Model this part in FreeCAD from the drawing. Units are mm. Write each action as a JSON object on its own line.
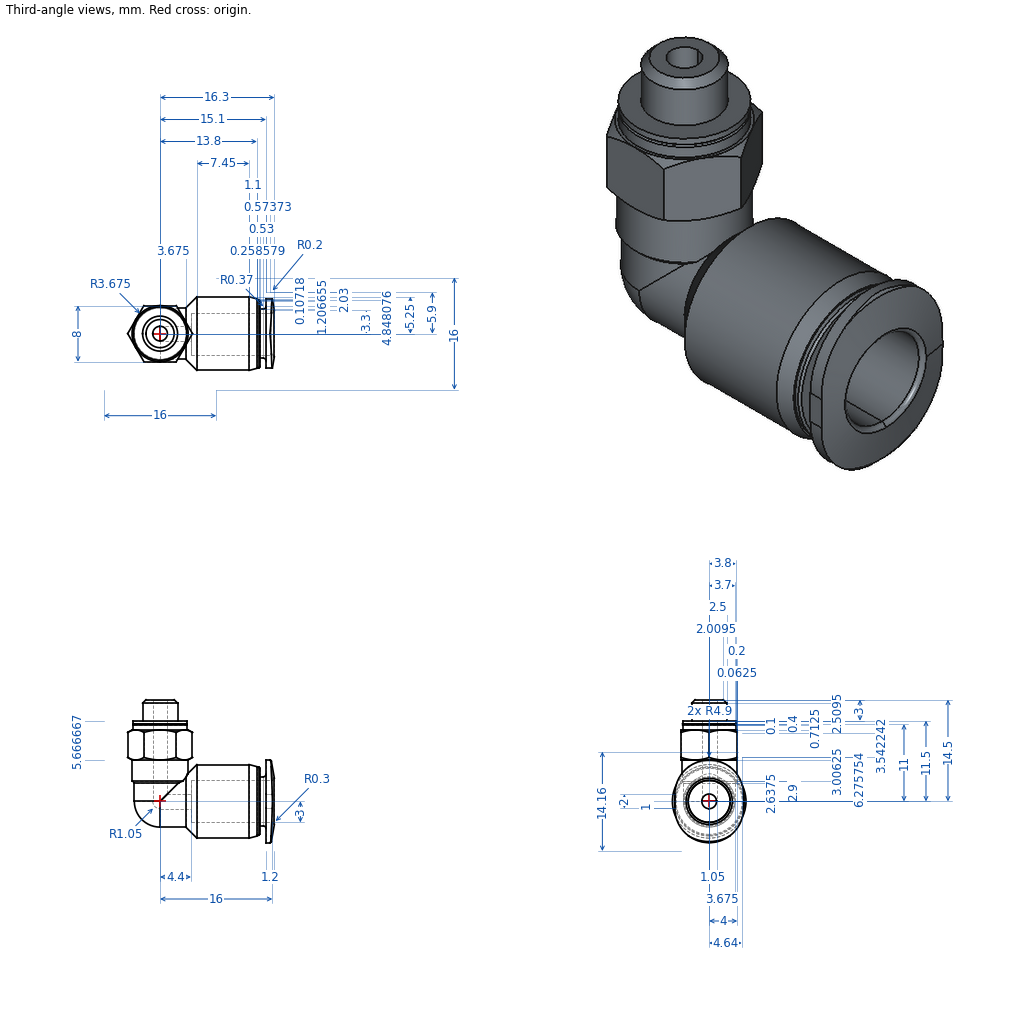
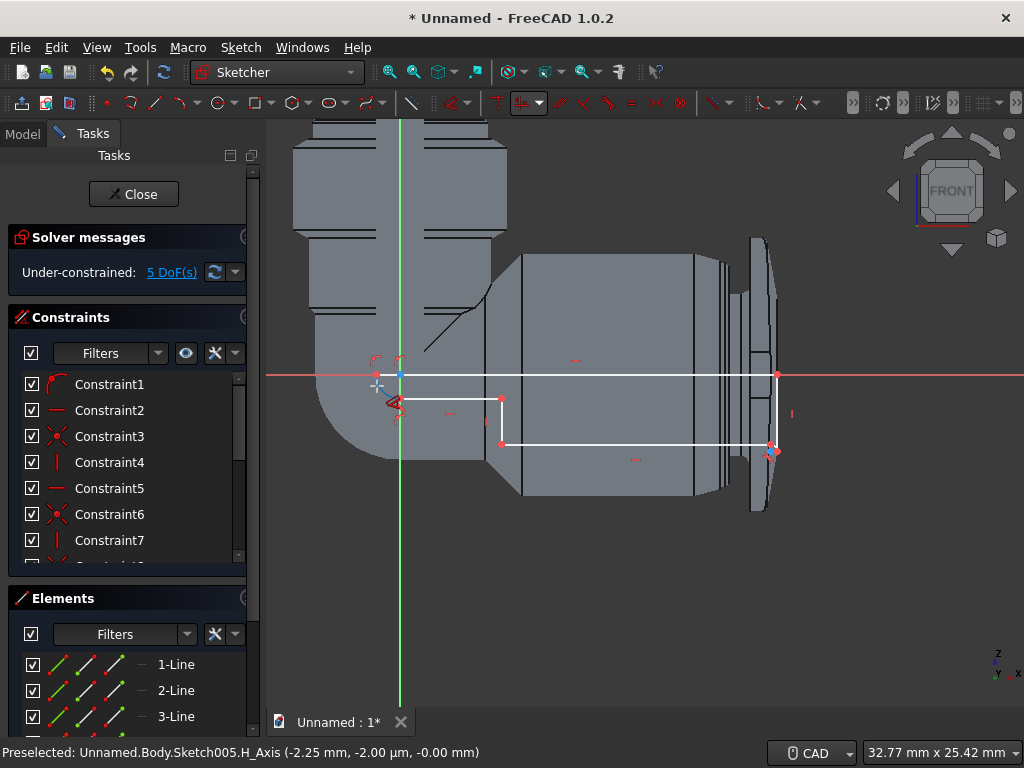
{"action": "scroll", "coordinate": [774, 445], "scroll_direction": "up", "scroll_amount": 9}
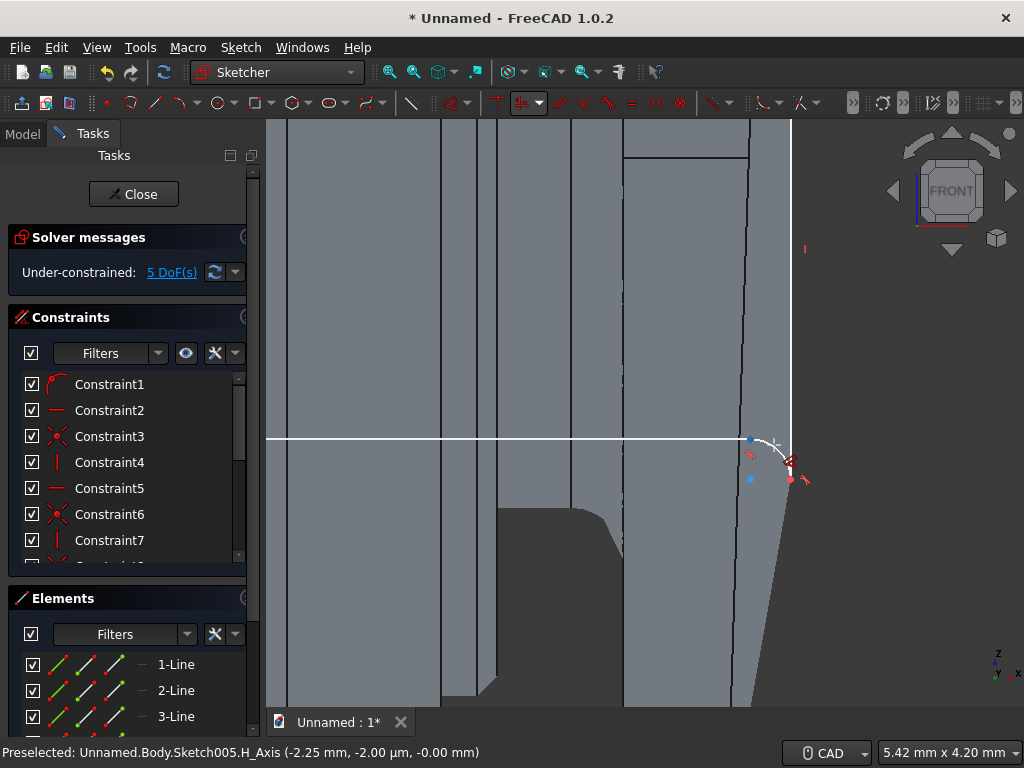
{"action": "left_click", "coordinate": [769, 444]}
{"action": "left_click", "coordinate": [810, 439]}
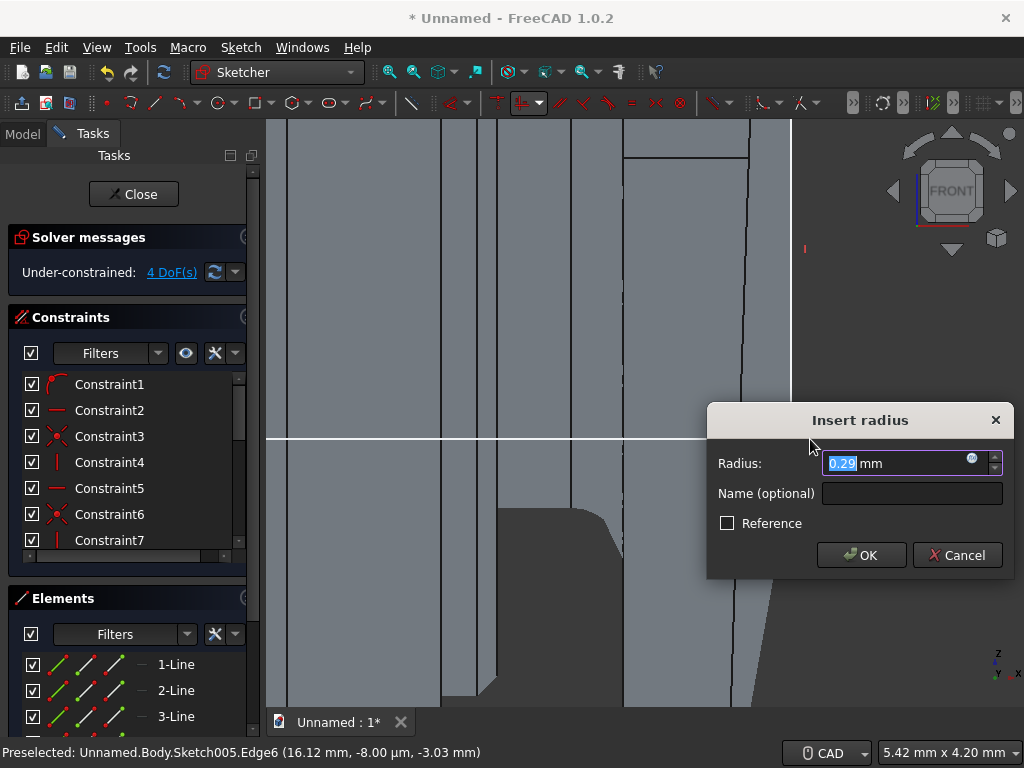
{"action": "type", "text": "0.3"}
{"action": "key", "text": "Return"}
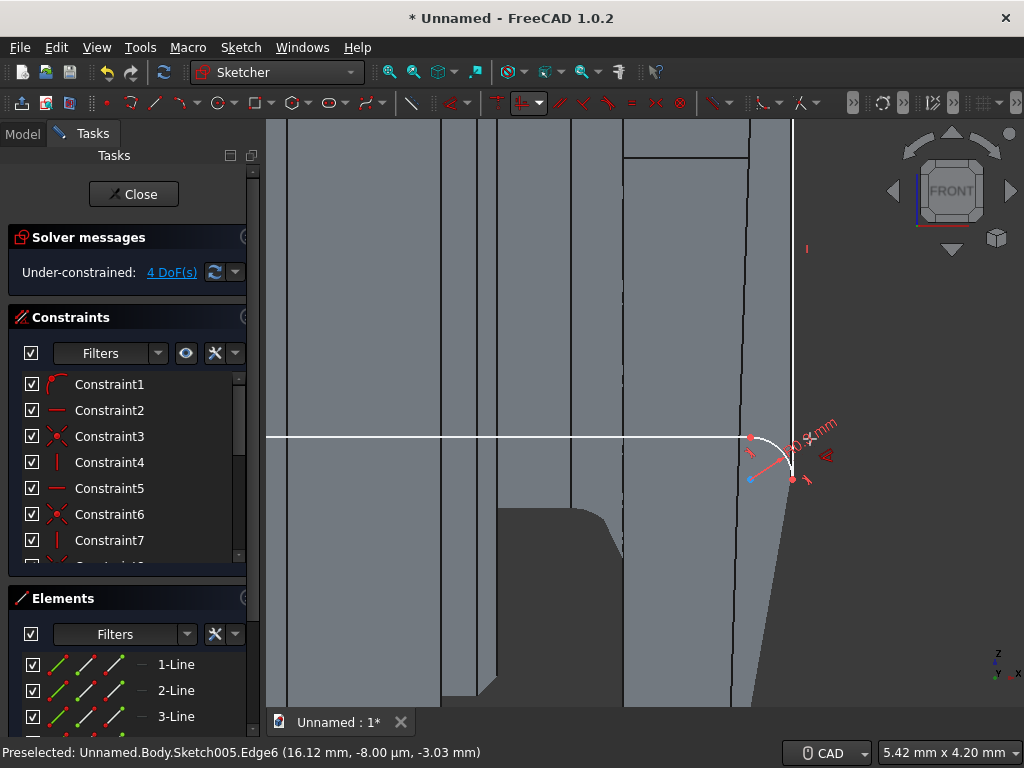
{"action": "scroll", "coordinate": [774, 445], "scroll_direction": "down", "scroll_amount": 9}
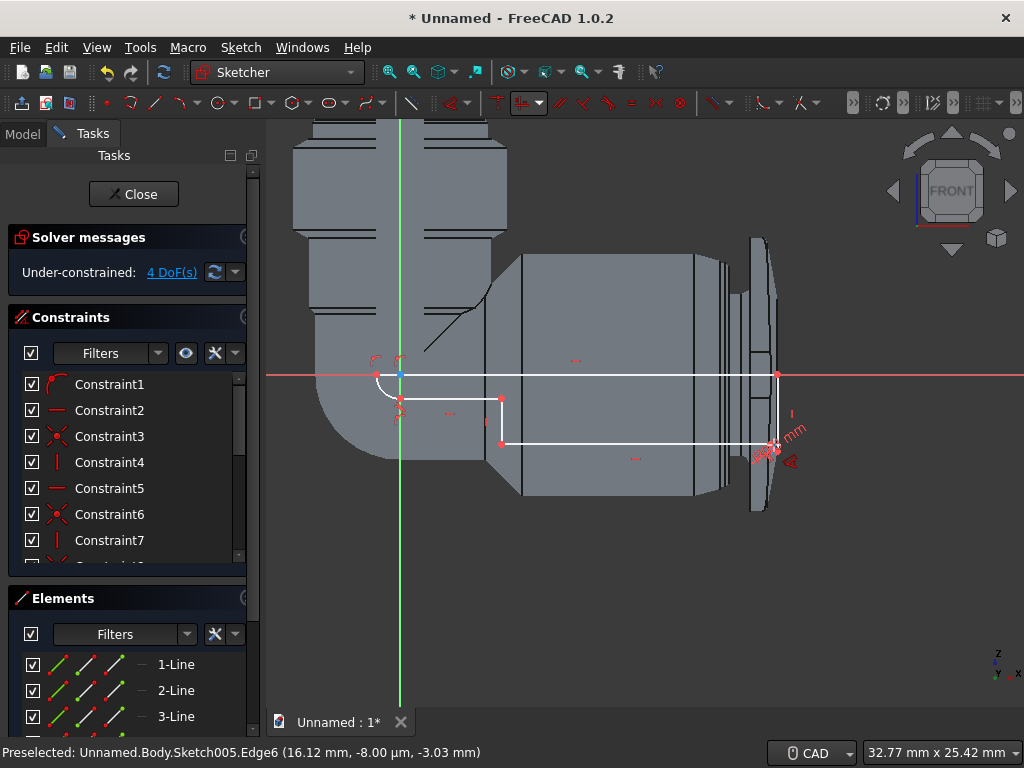
{"action": "scroll", "coordinate": [379, 386], "scroll_direction": "up", "scroll_amount": 3}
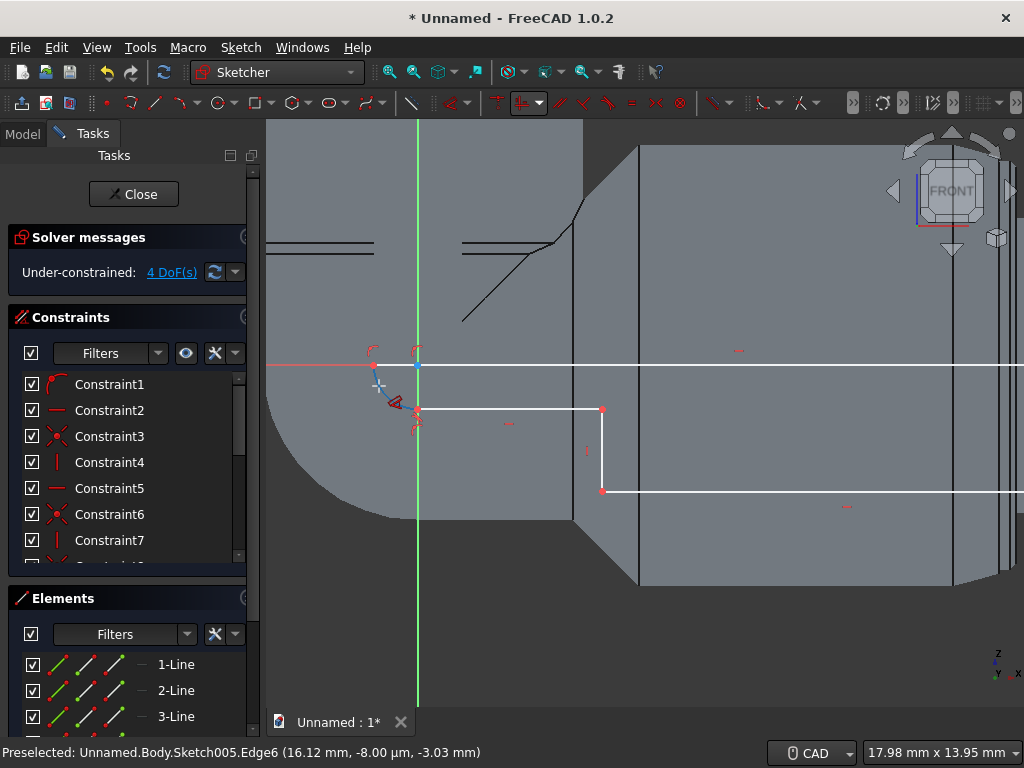
{"action": "left_click", "coordinate": [379, 385]}
{"action": "left_click", "coordinate": [350, 399]}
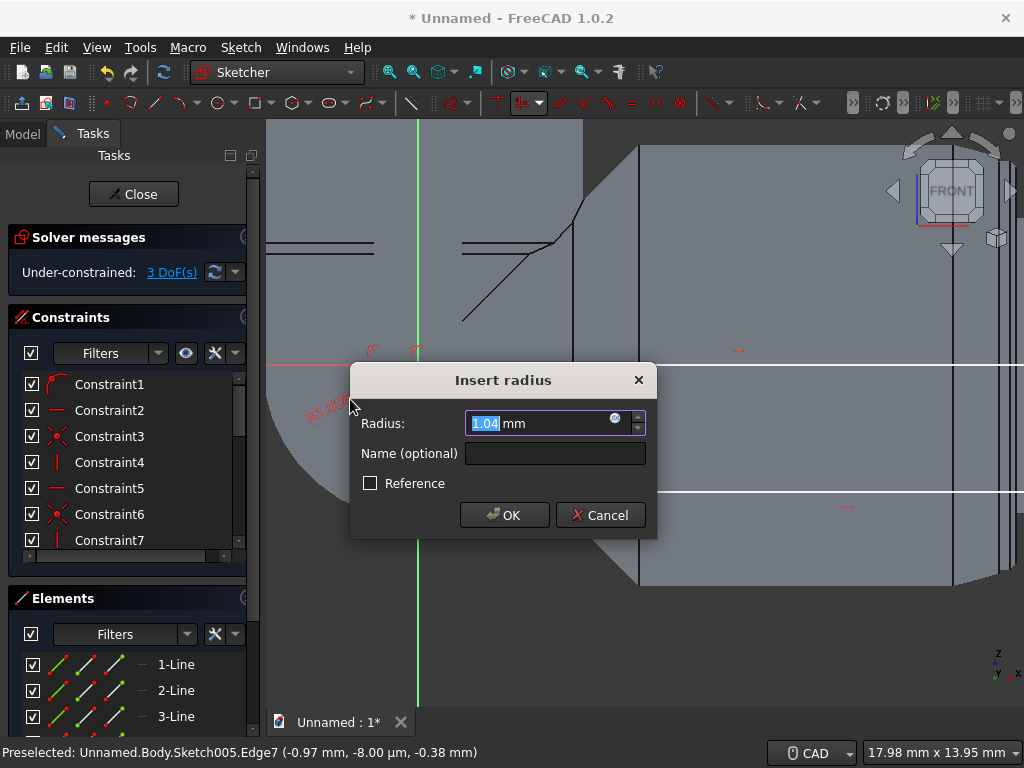
{"action": "type", "text": "1.05"}
{"action": "key", "text": "Return"}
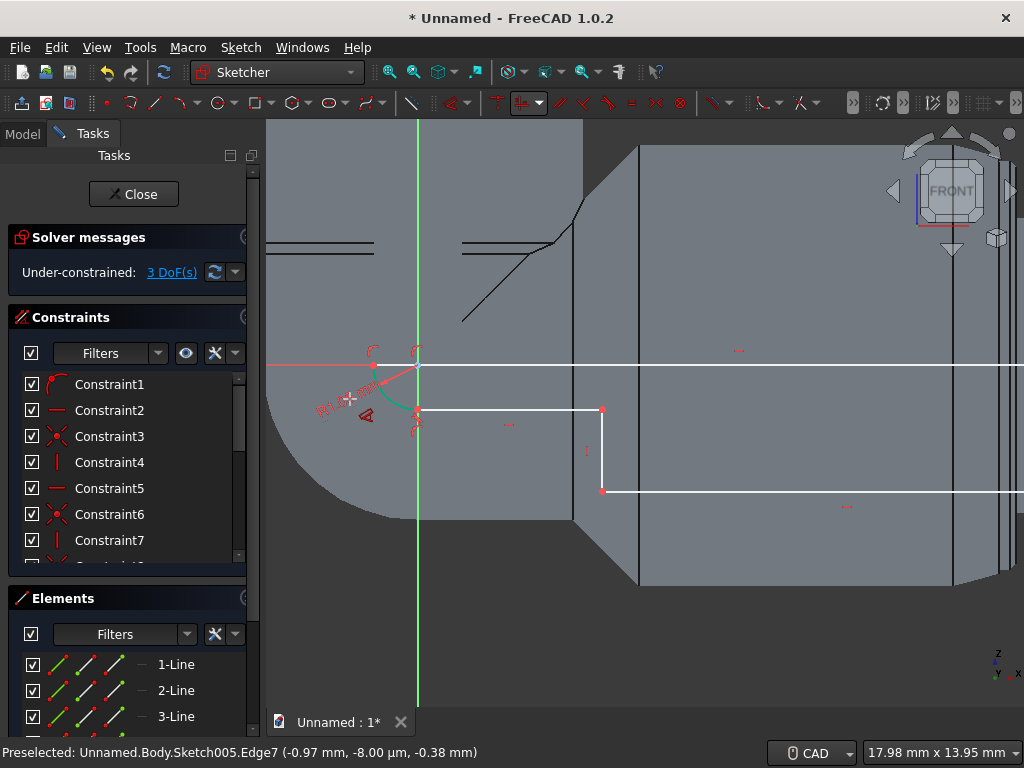
{"action": "scroll", "coordinate": [379, 386], "scroll_direction": "down", "scroll_amount": 3}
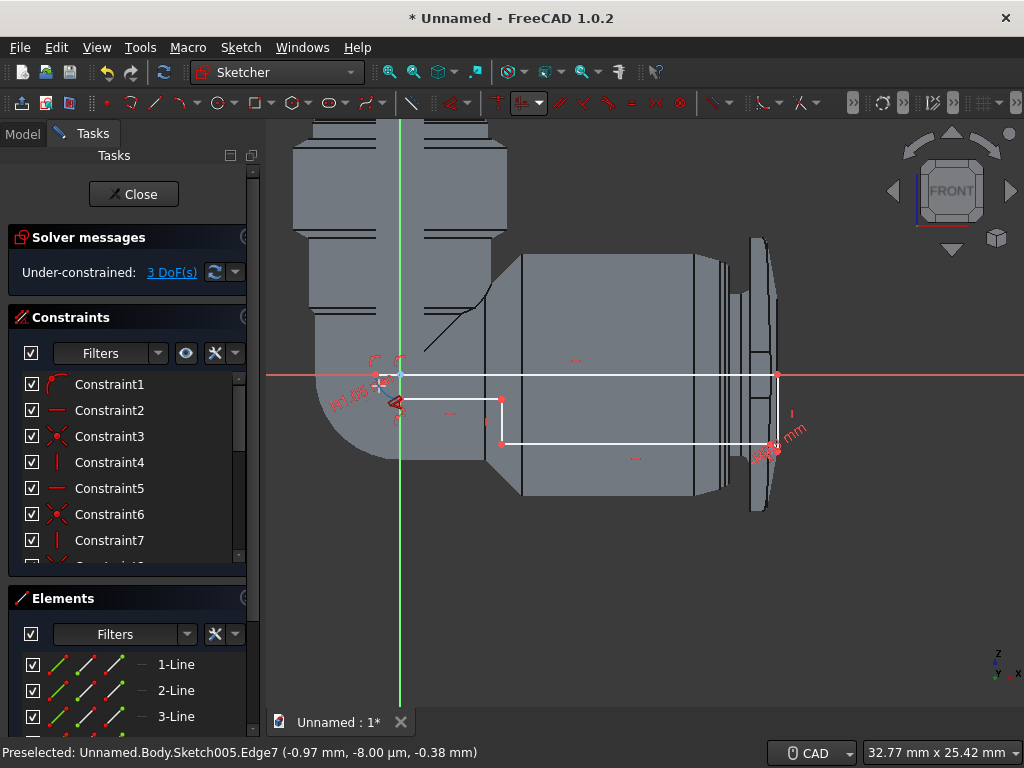
{"action": "scroll", "coordinate": [771, 444], "scroll_direction": "up", "scroll_amount": 3}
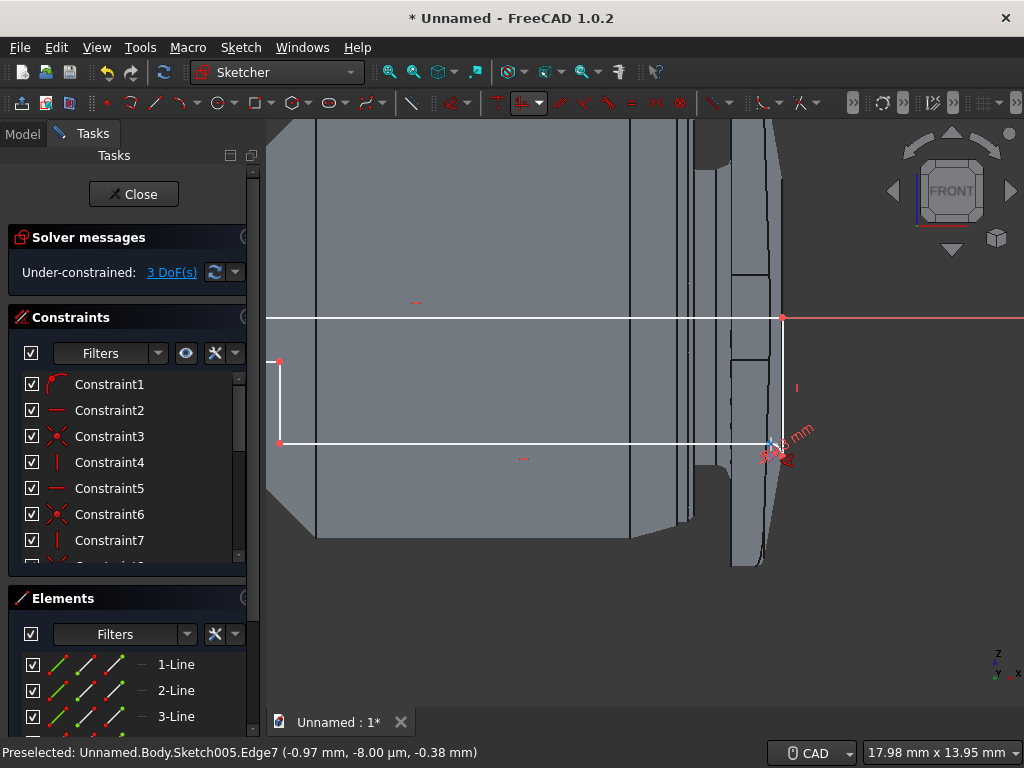
{"action": "left_click", "coordinate": [770, 444]}
{"action": "left_click", "coordinate": [804, 381]}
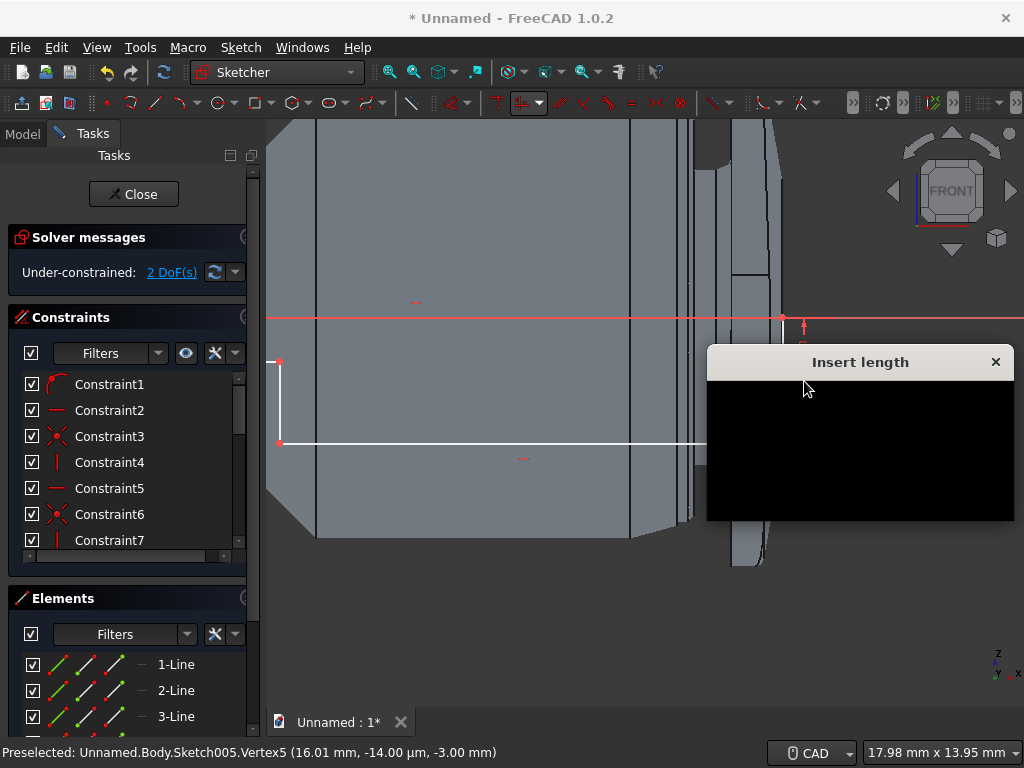
{"action": "type", "text": "3"}
{"action": "key", "text": "Return"}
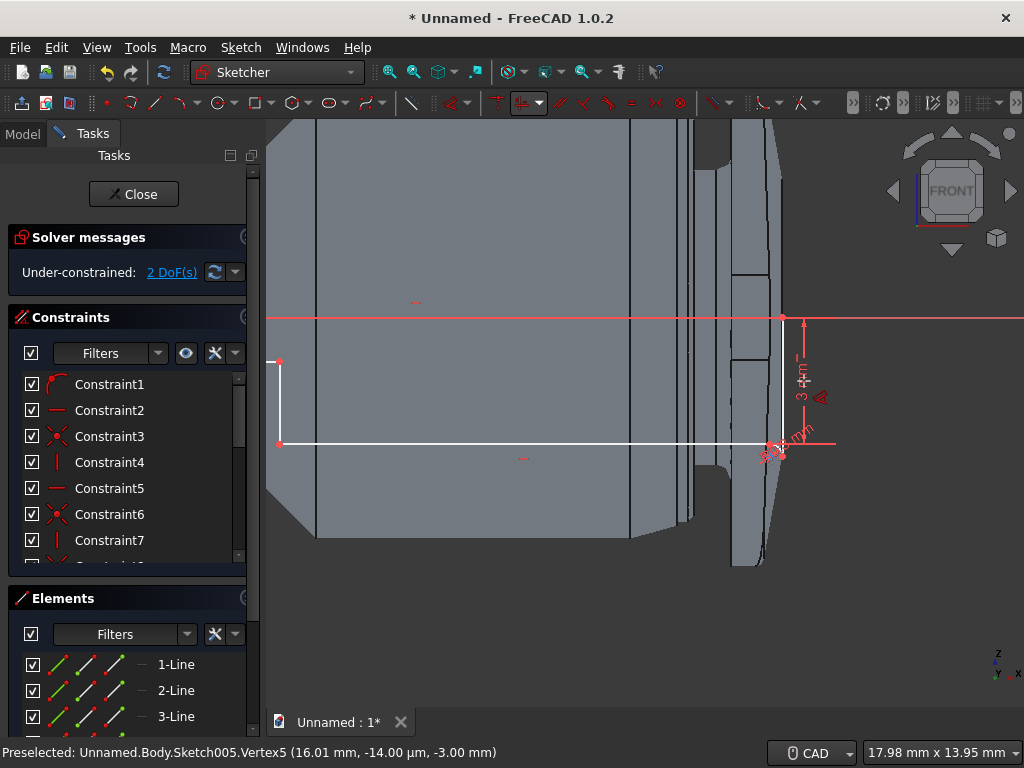
{"action": "scroll", "coordinate": [771, 444], "scroll_direction": "down", "scroll_amount": 3}